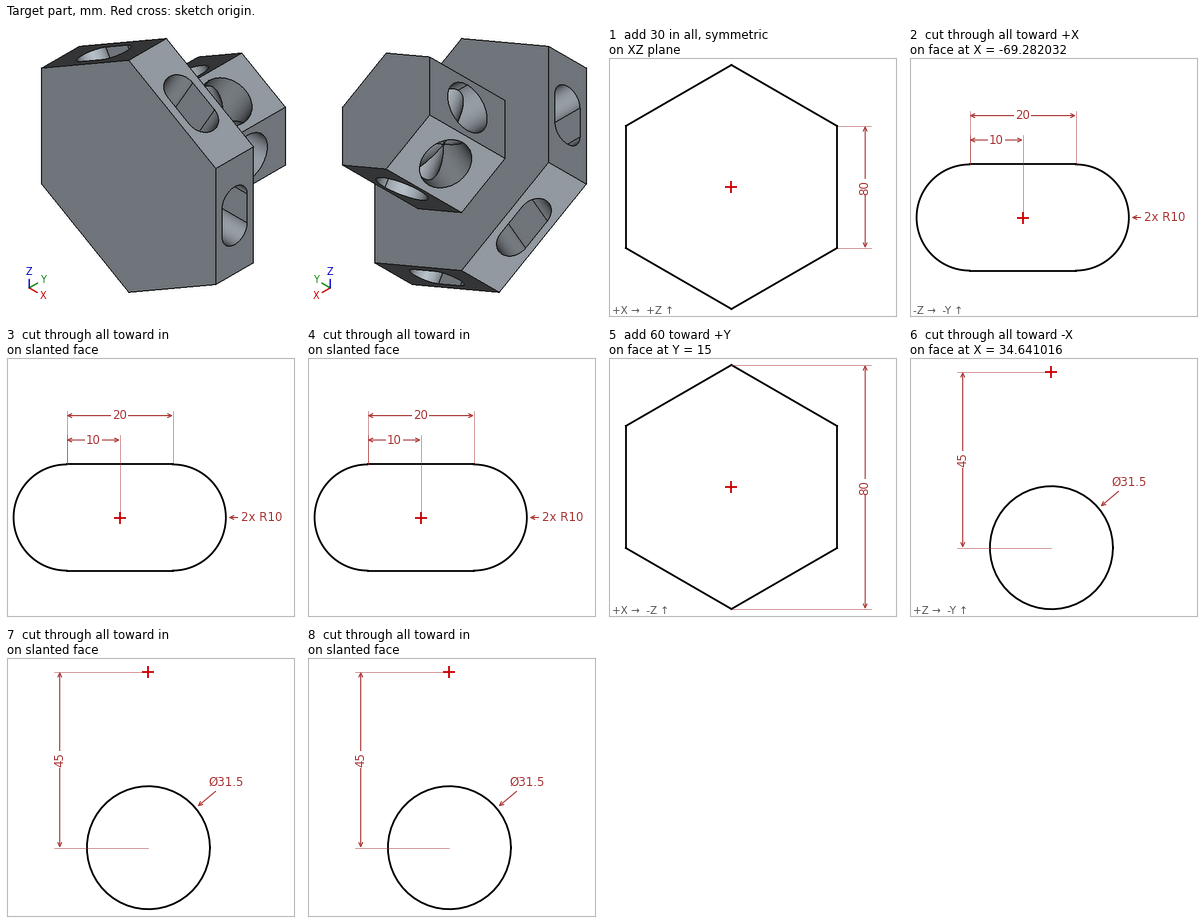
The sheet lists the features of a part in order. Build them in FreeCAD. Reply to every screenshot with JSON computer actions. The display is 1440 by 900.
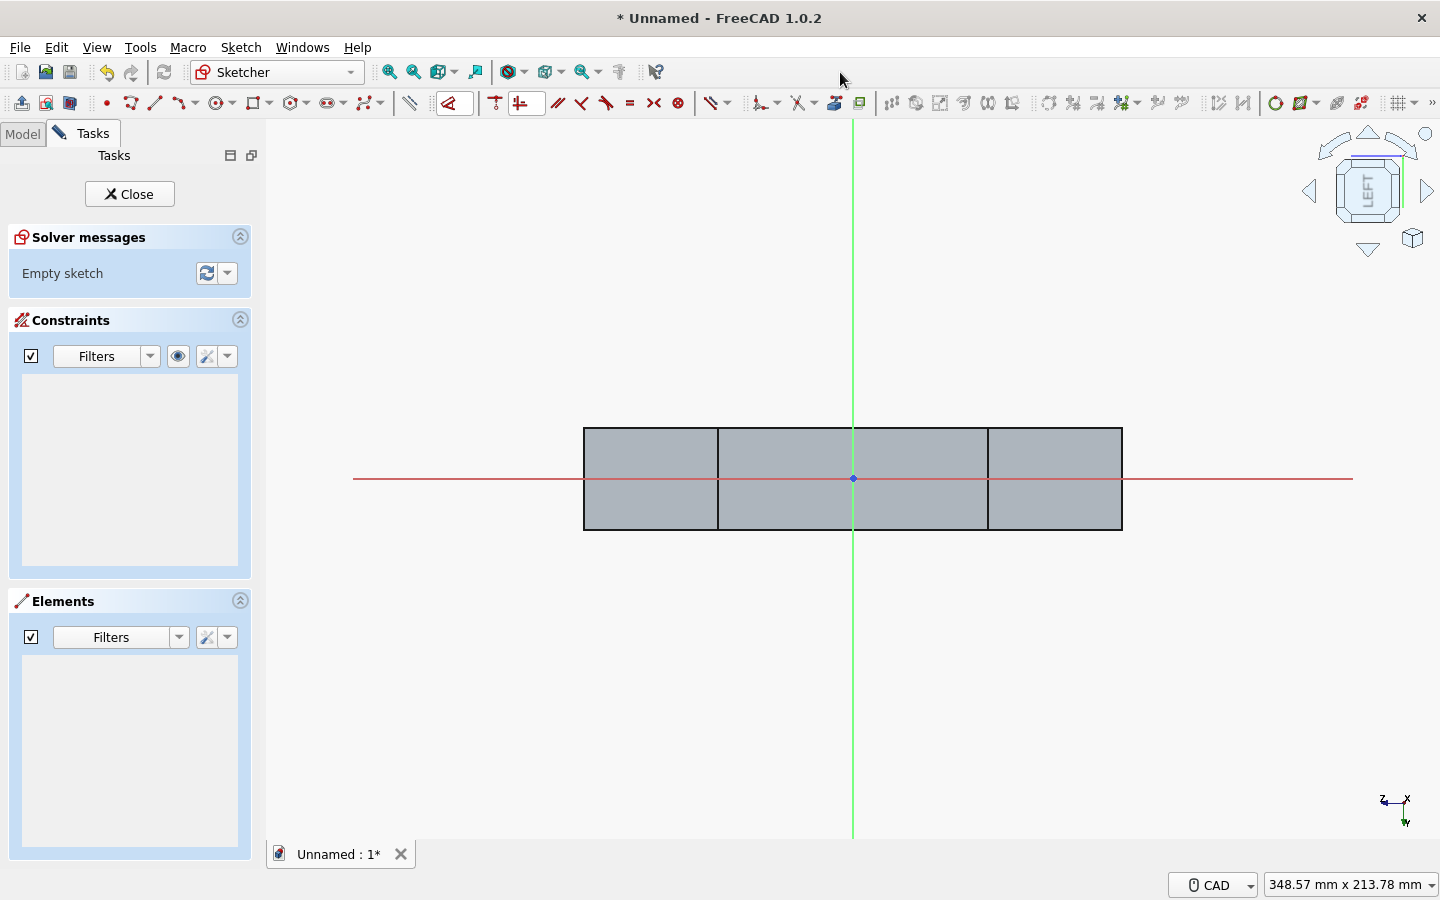
{"action": "scroll", "coordinate": [870, 479], "scroll_direction": "up", "scroll_amount": 8}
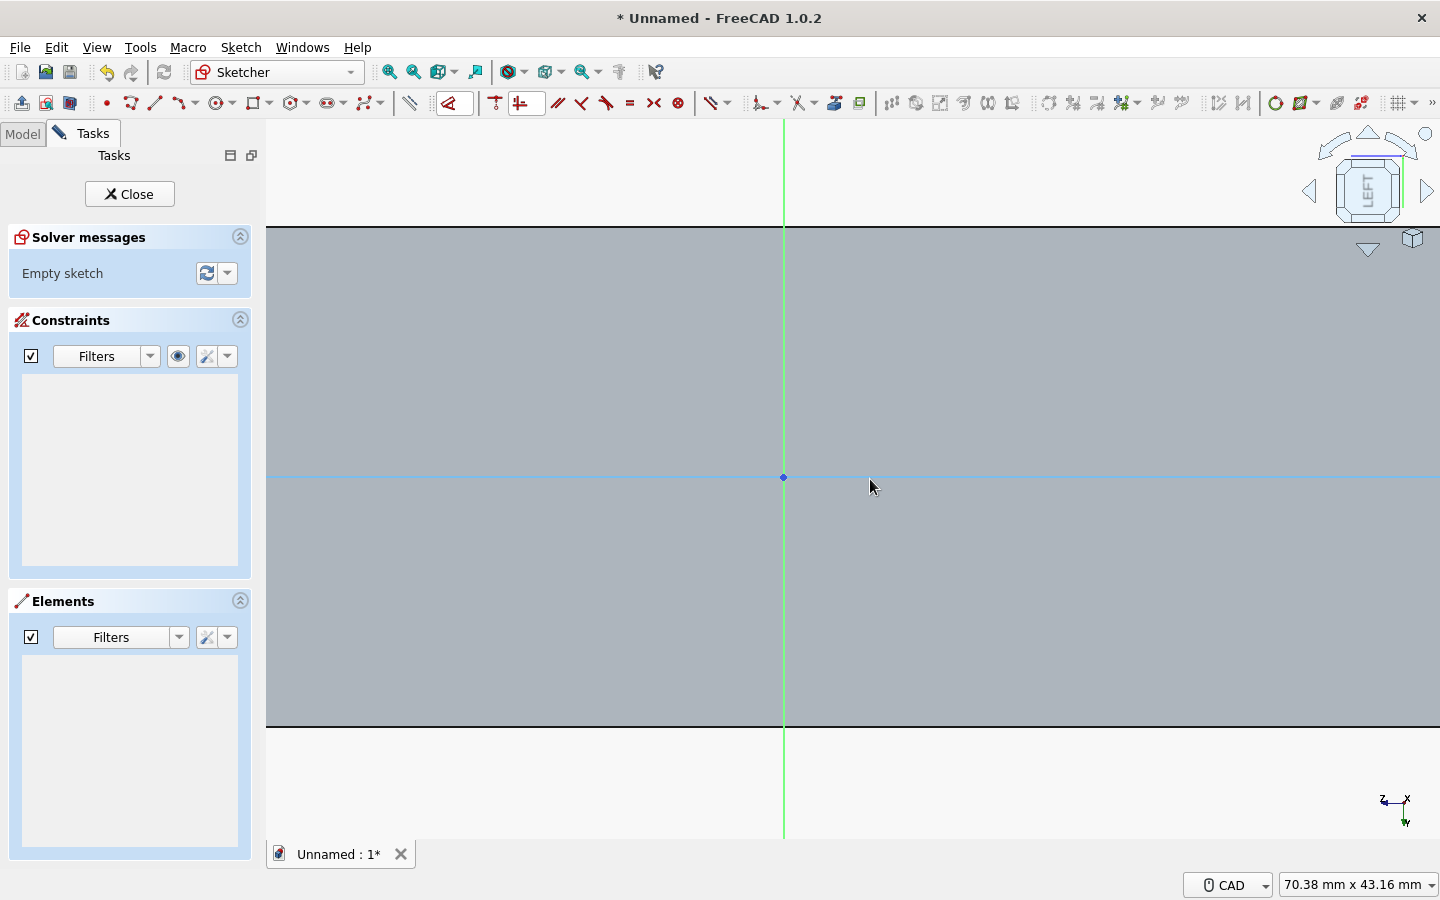
{"action": "left_click", "coordinate": [328, 104]}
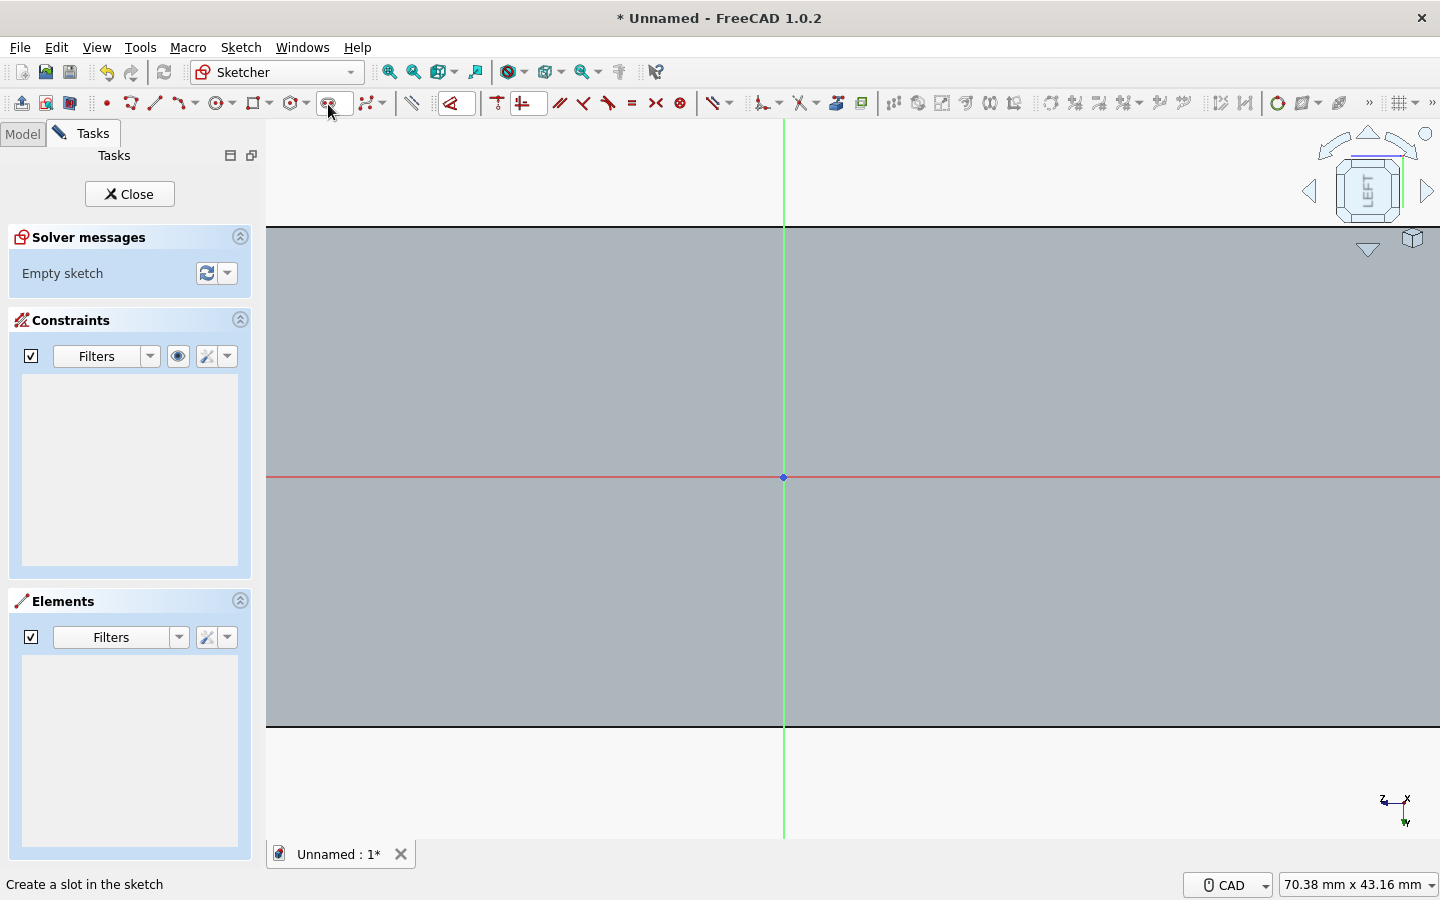
{"action": "left_click", "coordinate": [617, 477]}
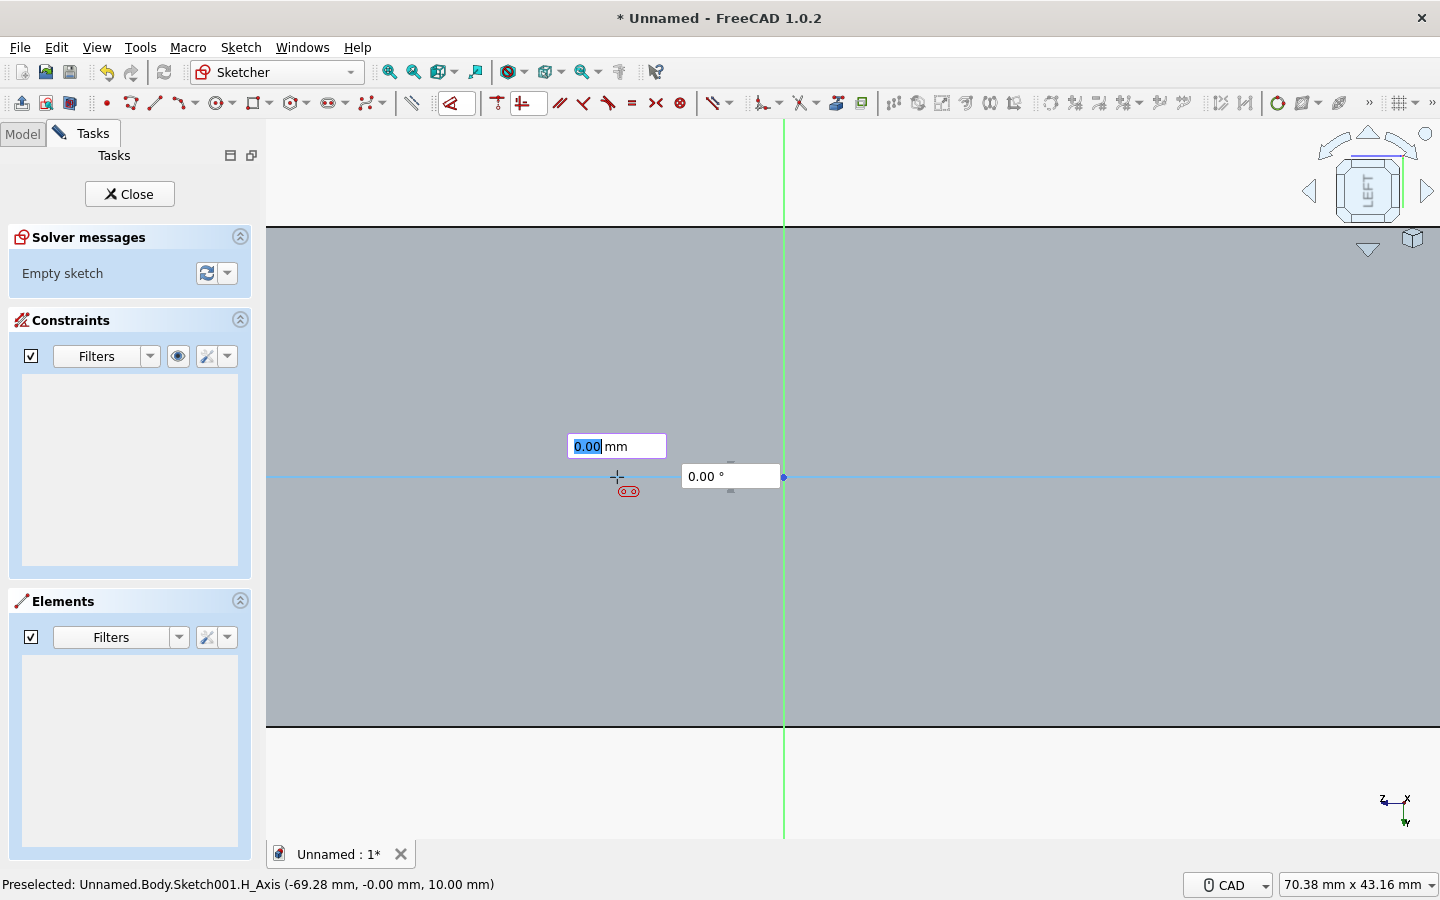
{"action": "left_click", "coordinate": [951, 468]}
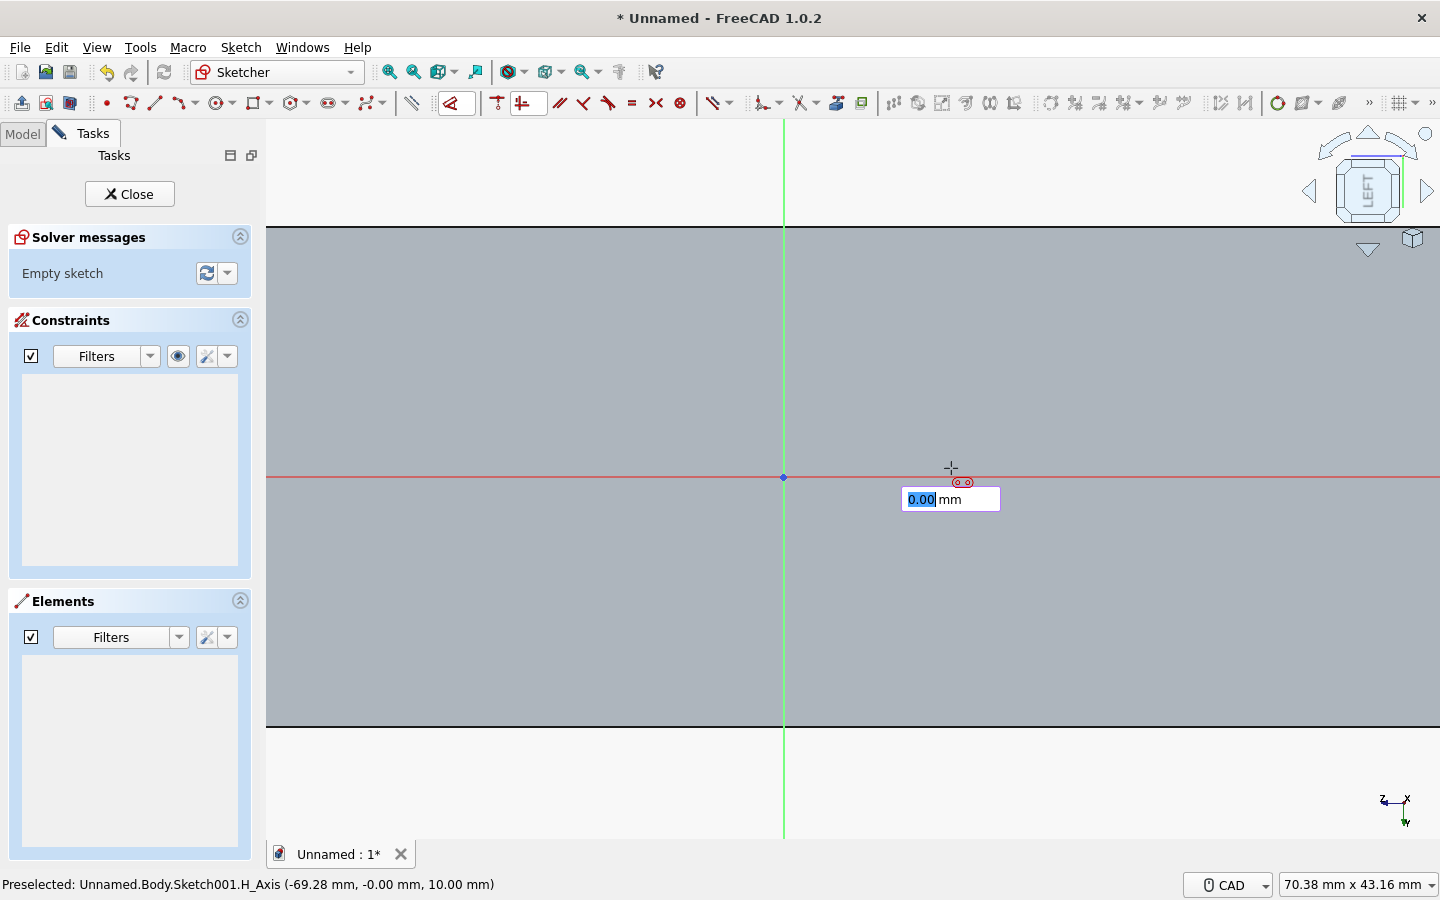
{"action": "left_click", "coordinate": [734, 644]}
{"action": "key", "text": "Escape"}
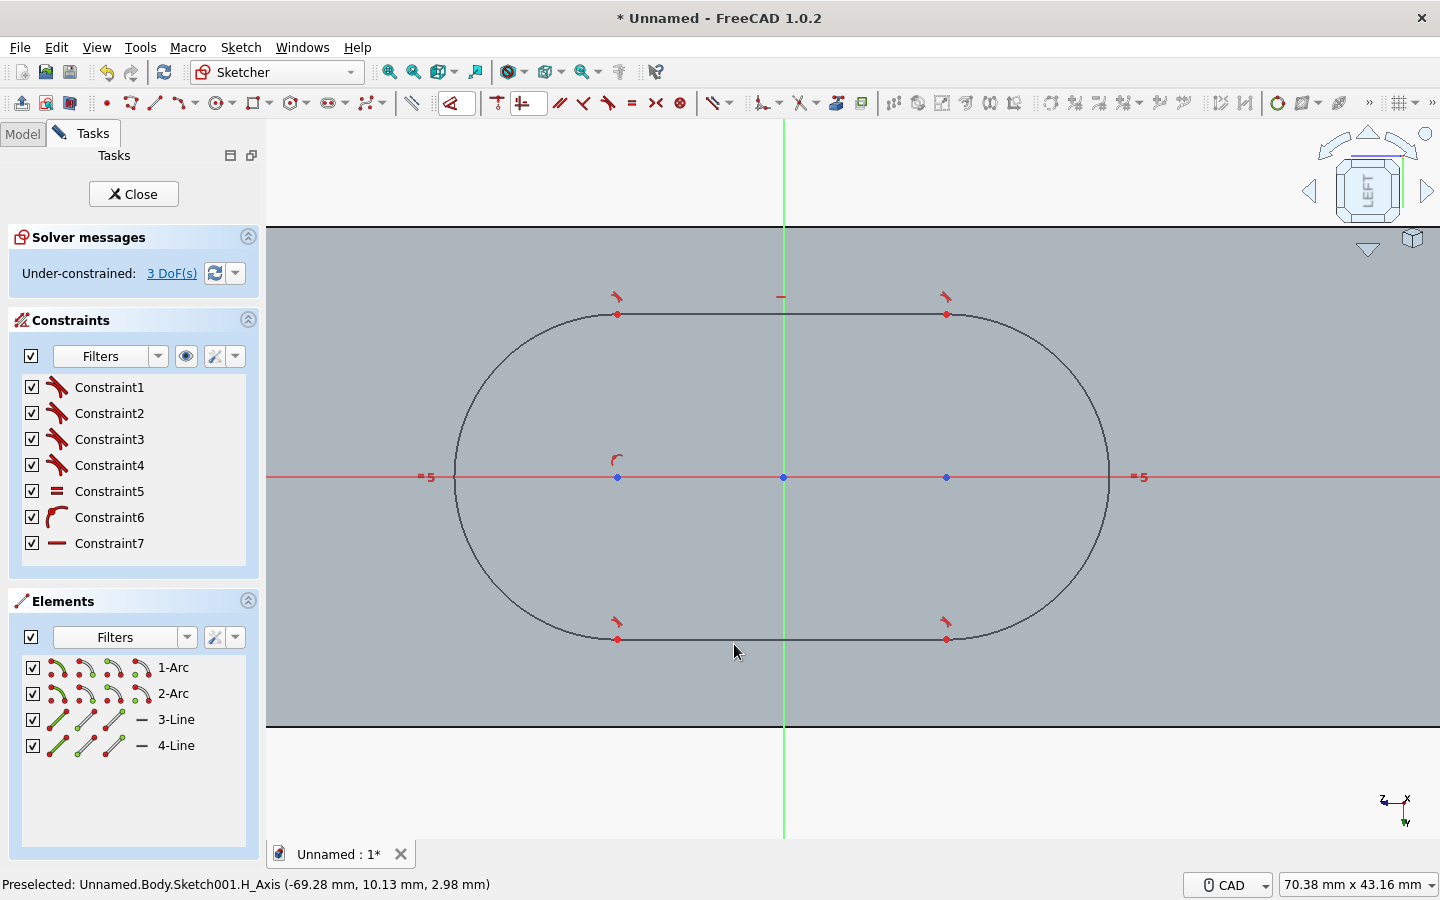
{"action": "left_click", "coordinate": [486, 381]}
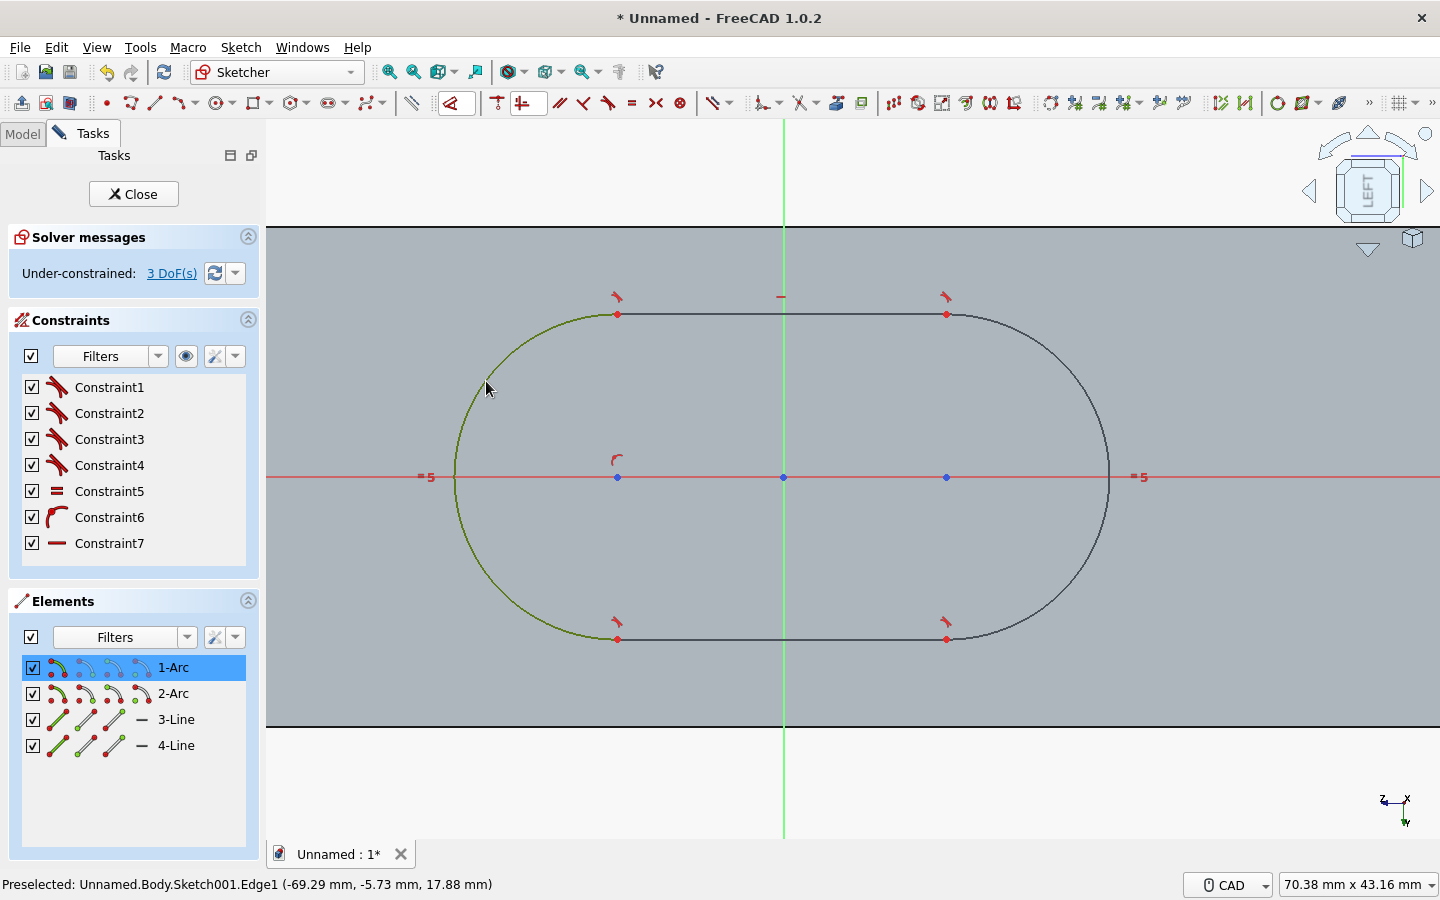
{"action": "left_click", "coordinate": [470, 104]}